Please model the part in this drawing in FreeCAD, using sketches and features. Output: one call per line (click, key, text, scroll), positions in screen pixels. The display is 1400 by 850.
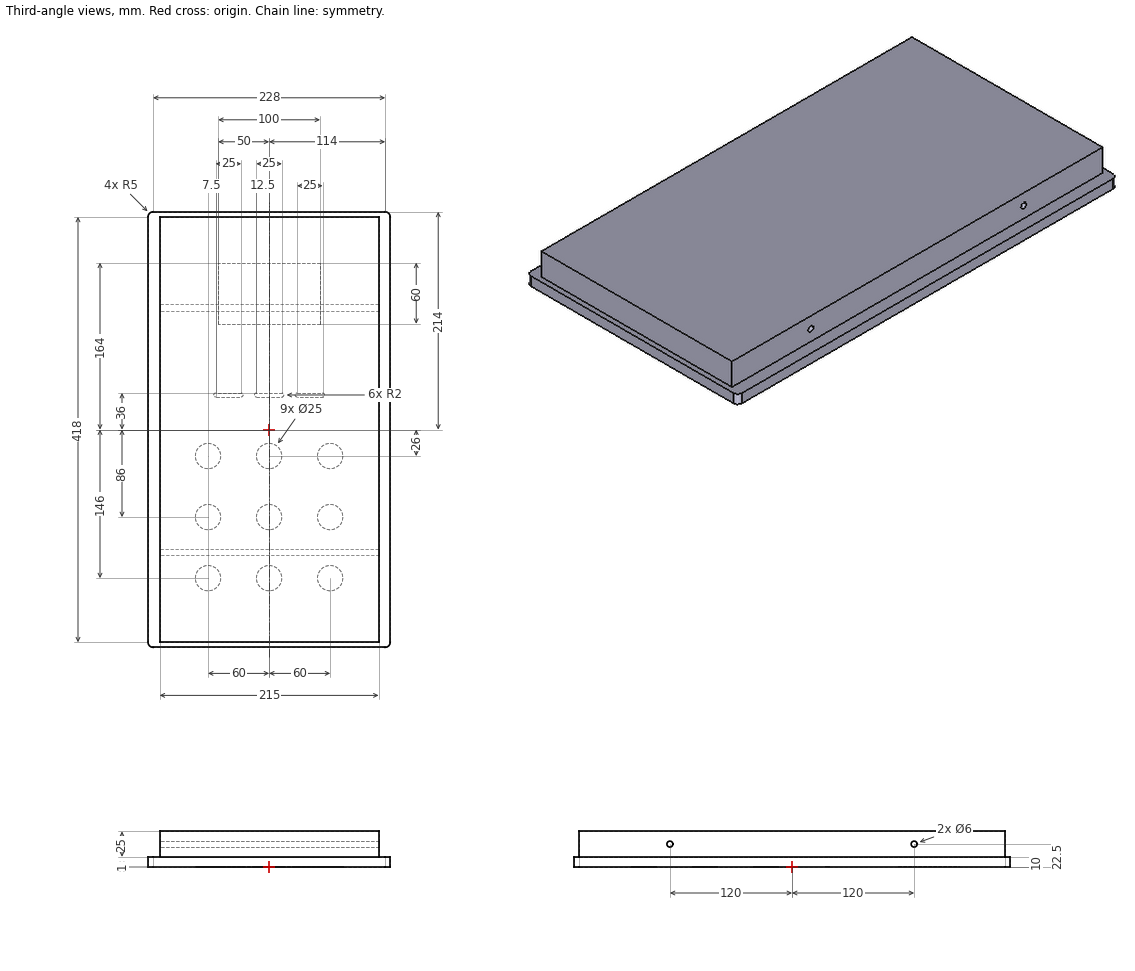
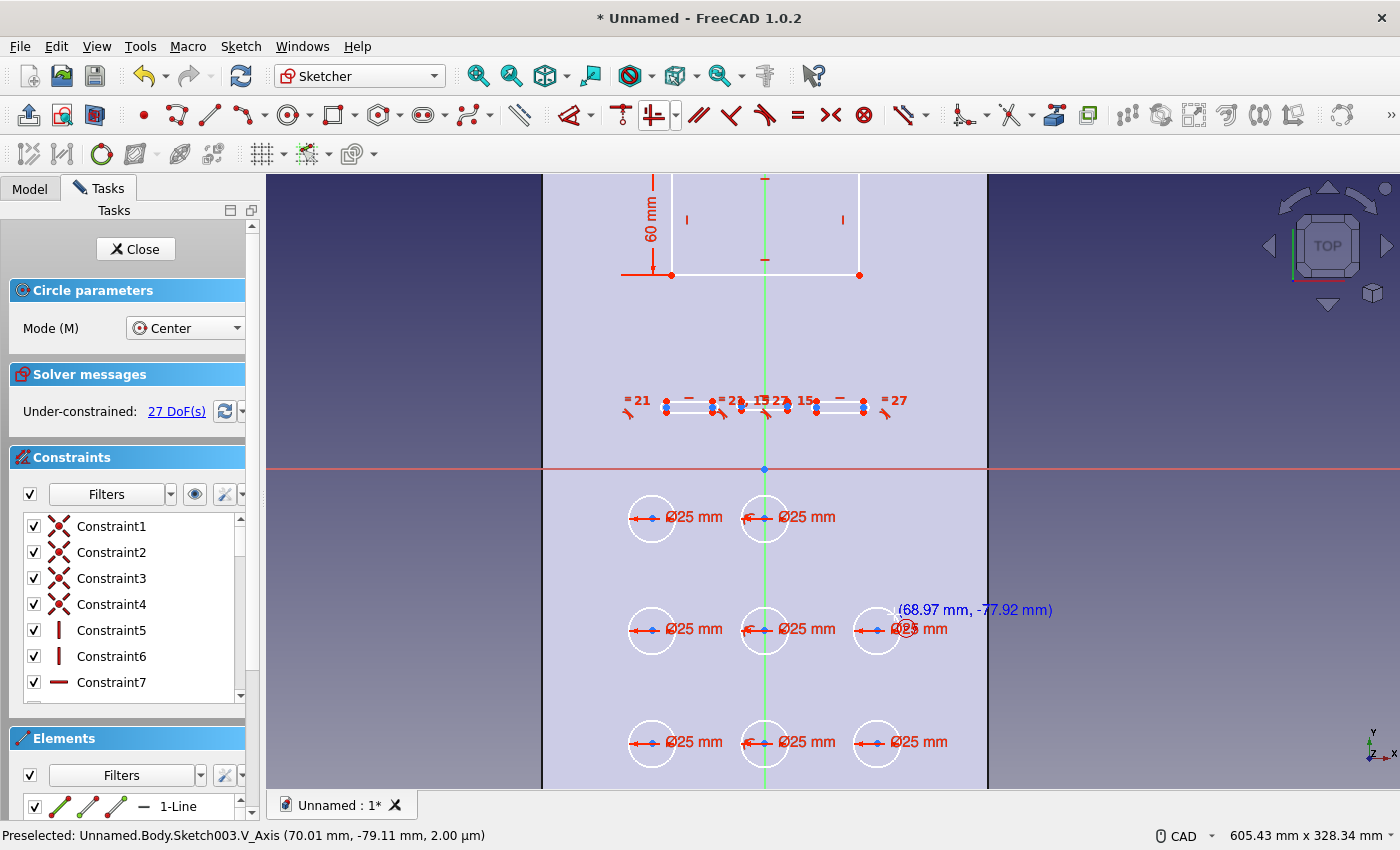
click(877, 518)
move(894, 501)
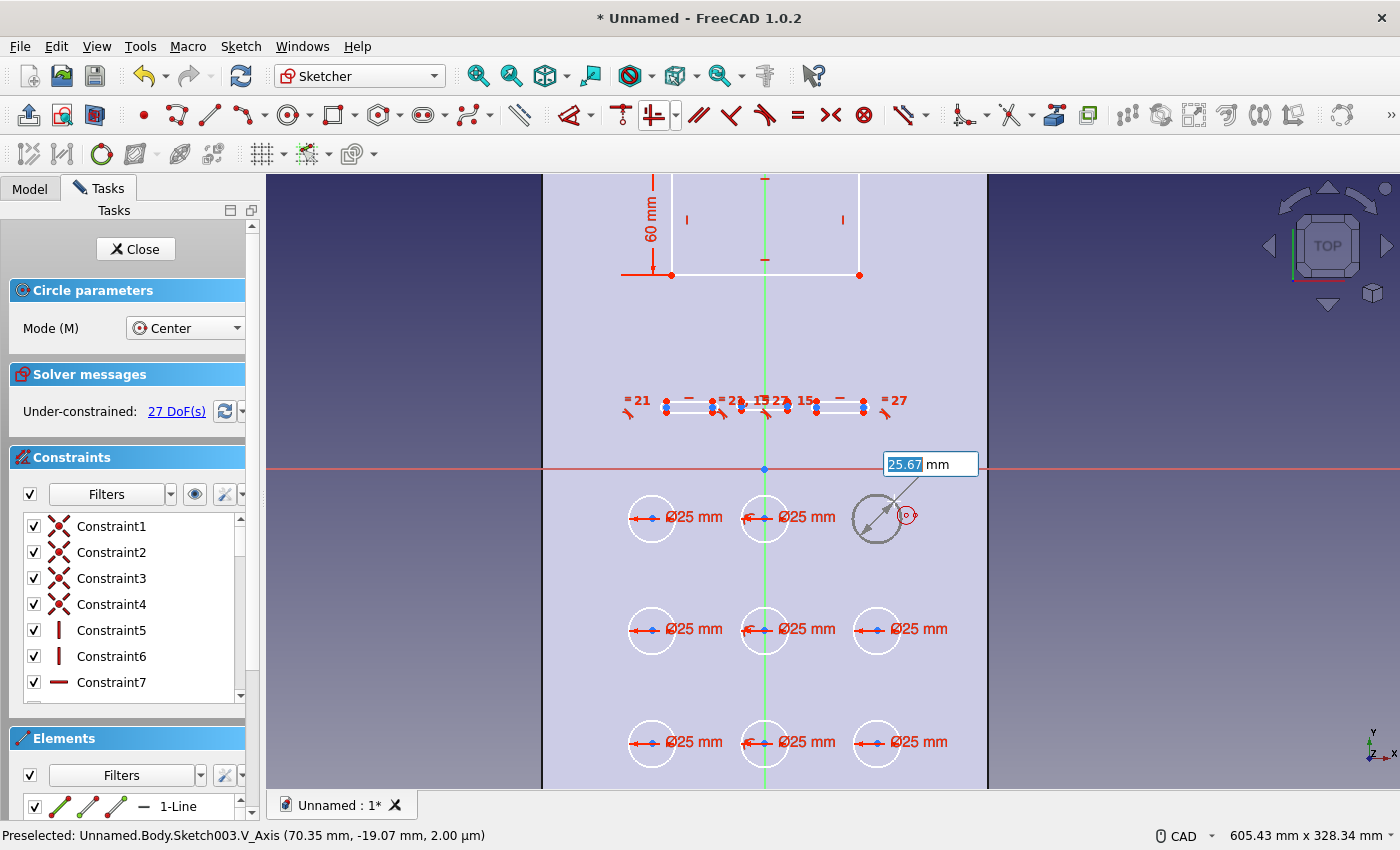
text(25)
key(Return)
key(Escape)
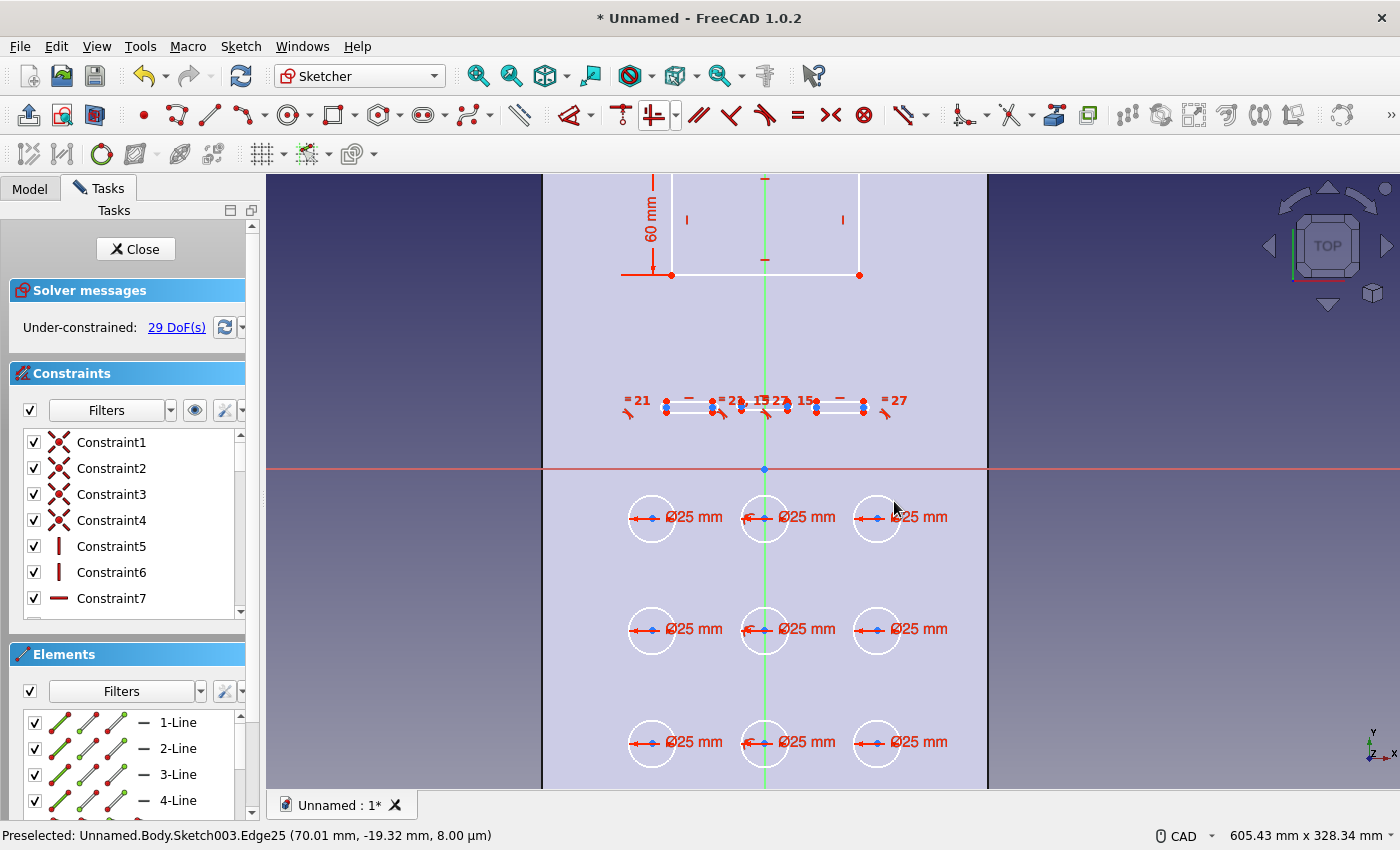
scroll(737, 406, up, 6)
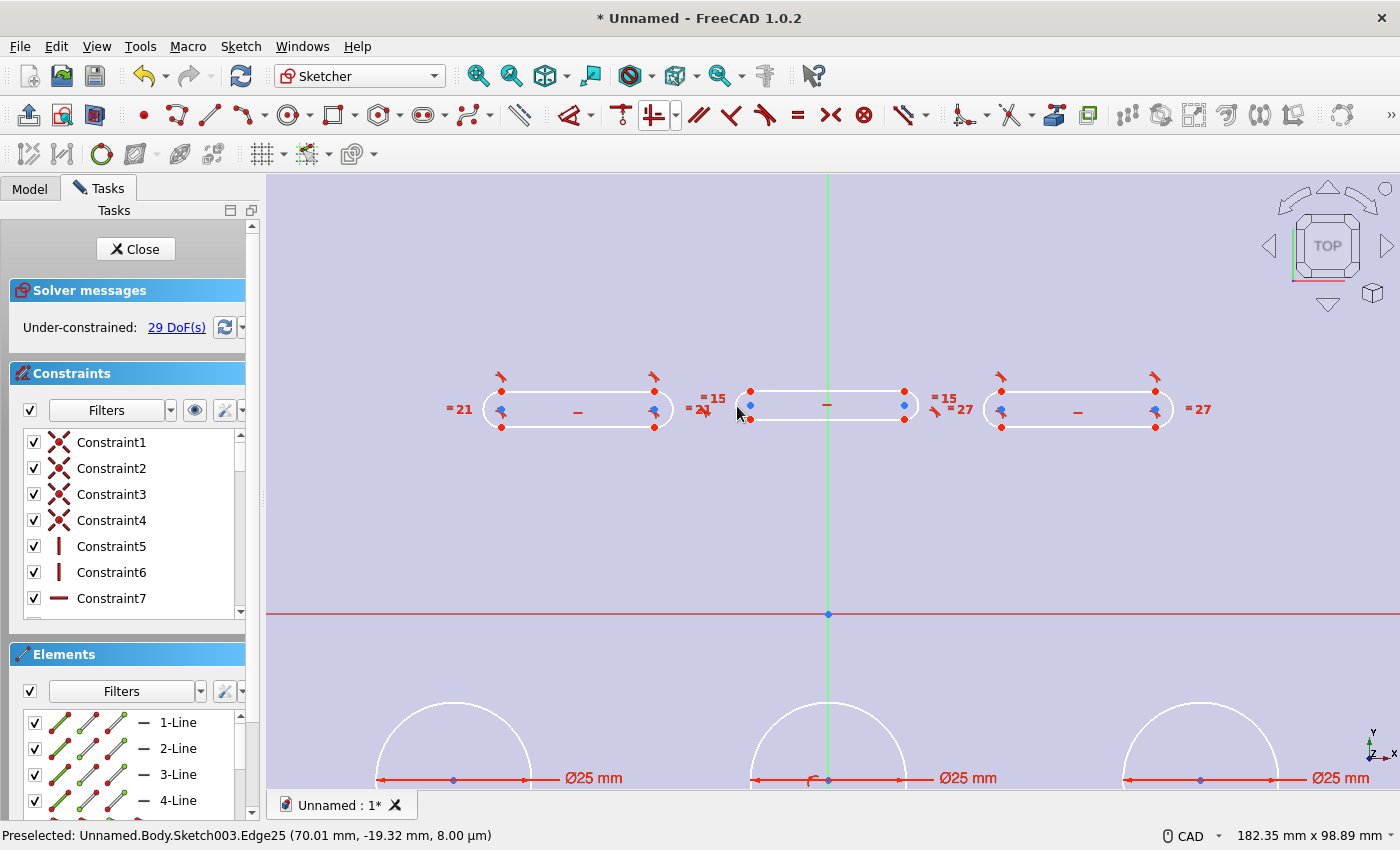
click(736, 406)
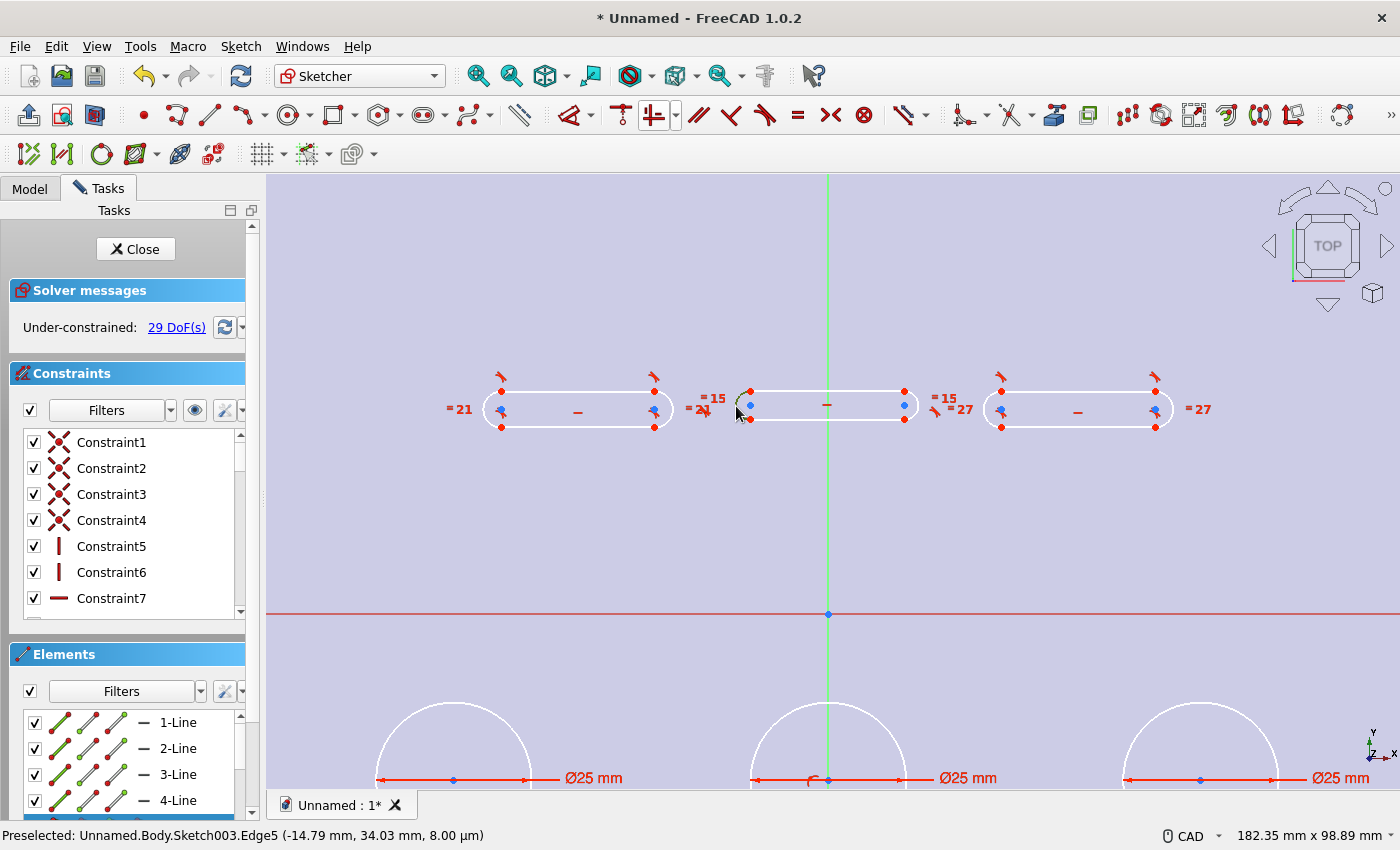
click(487, 399)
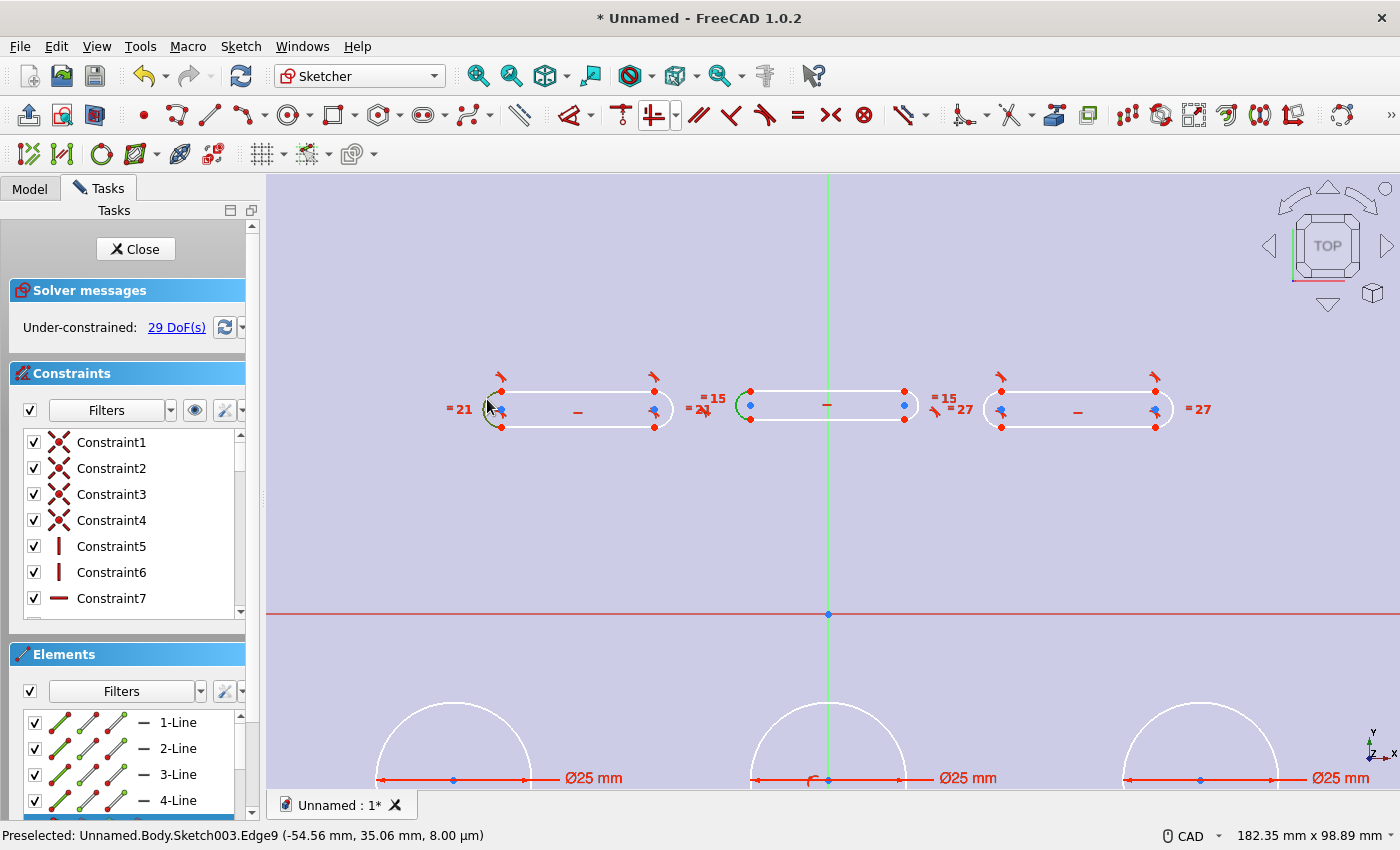
click(987, 399)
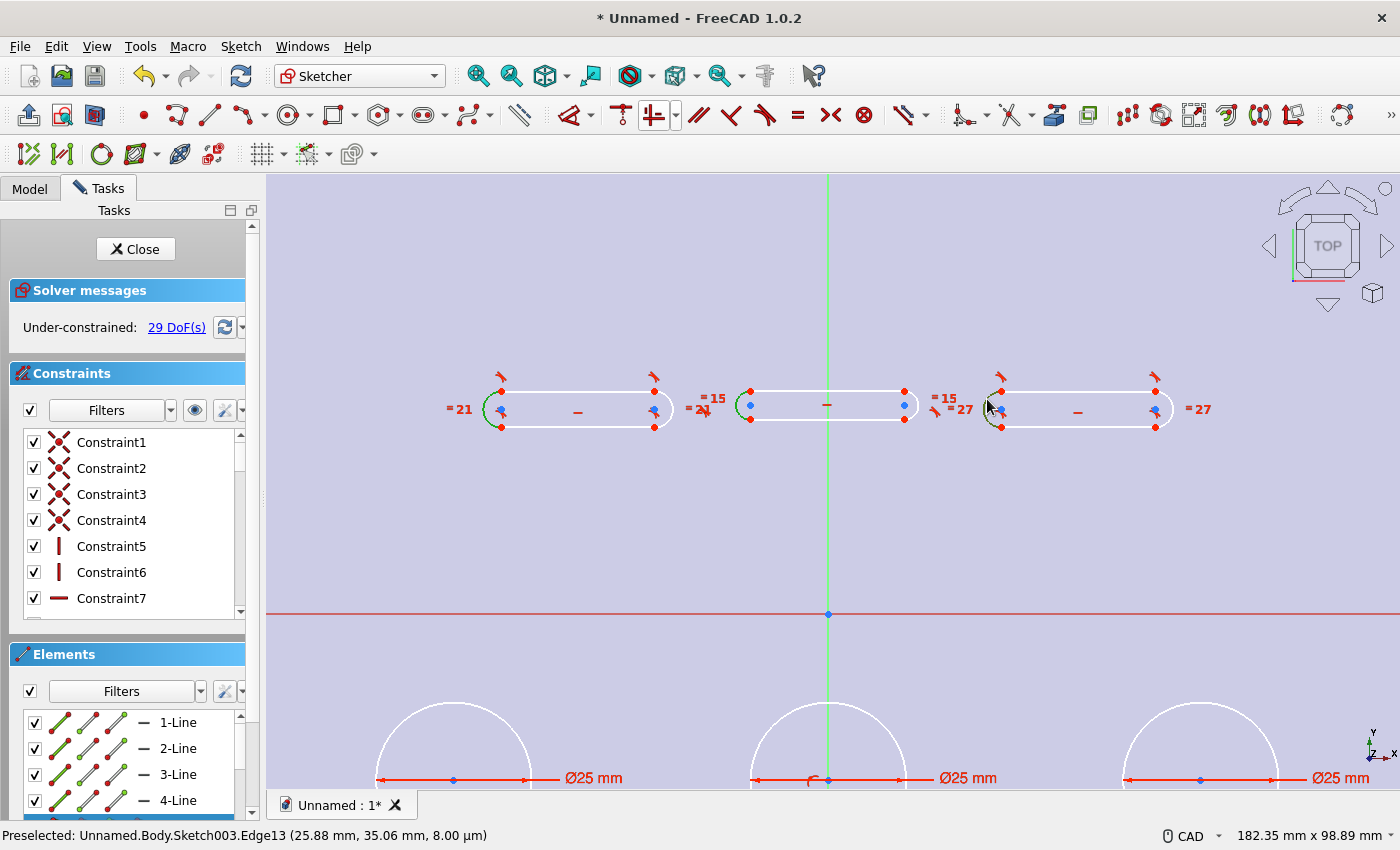
click(798, 116)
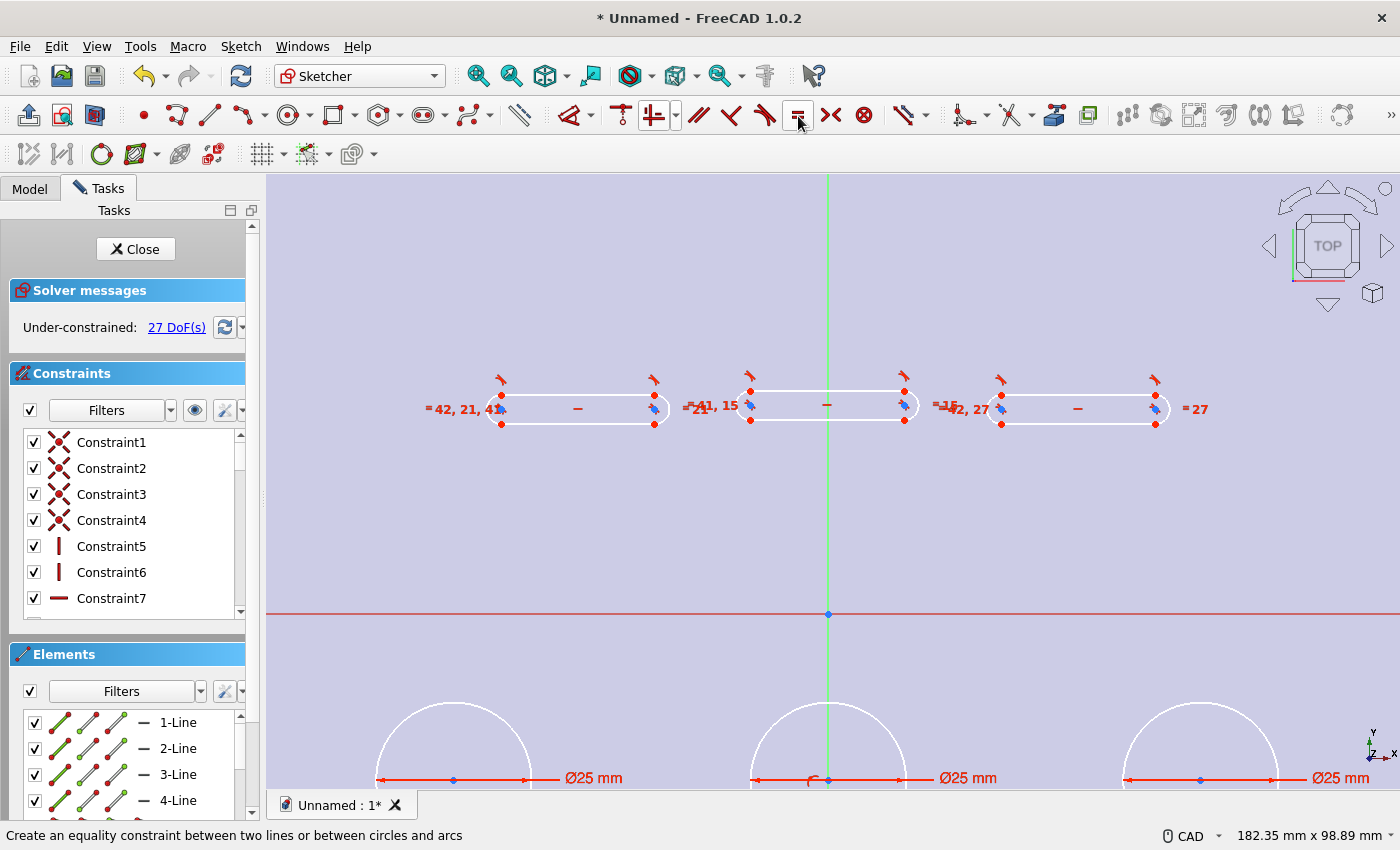
scroll(748, 452, down, 8)